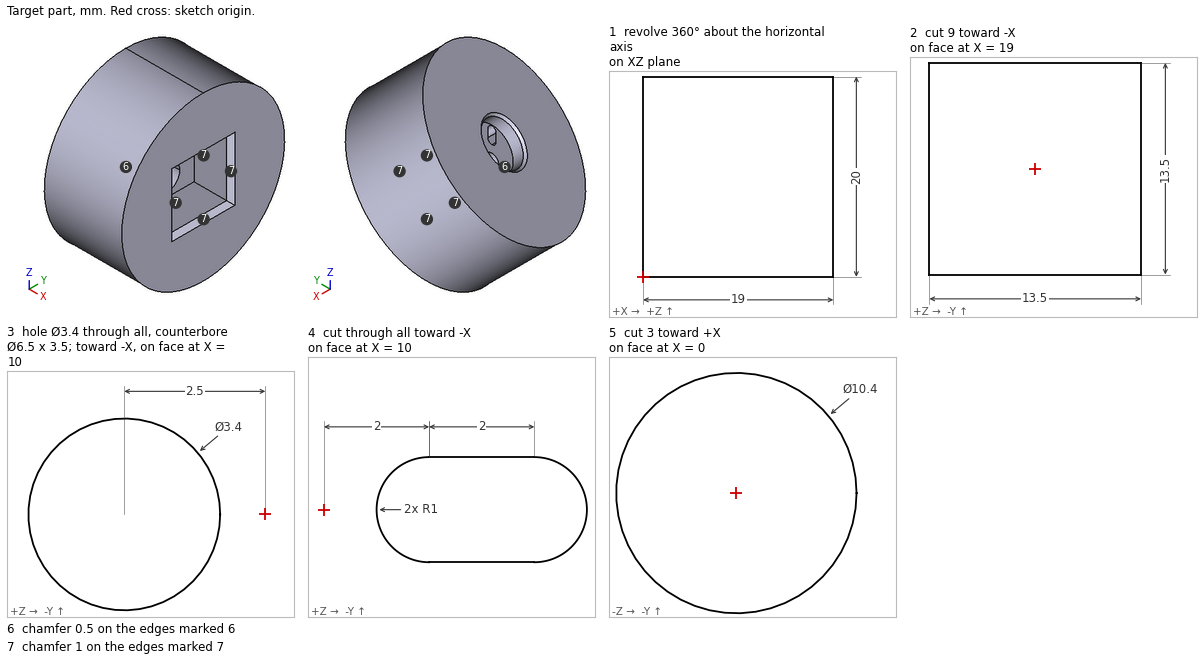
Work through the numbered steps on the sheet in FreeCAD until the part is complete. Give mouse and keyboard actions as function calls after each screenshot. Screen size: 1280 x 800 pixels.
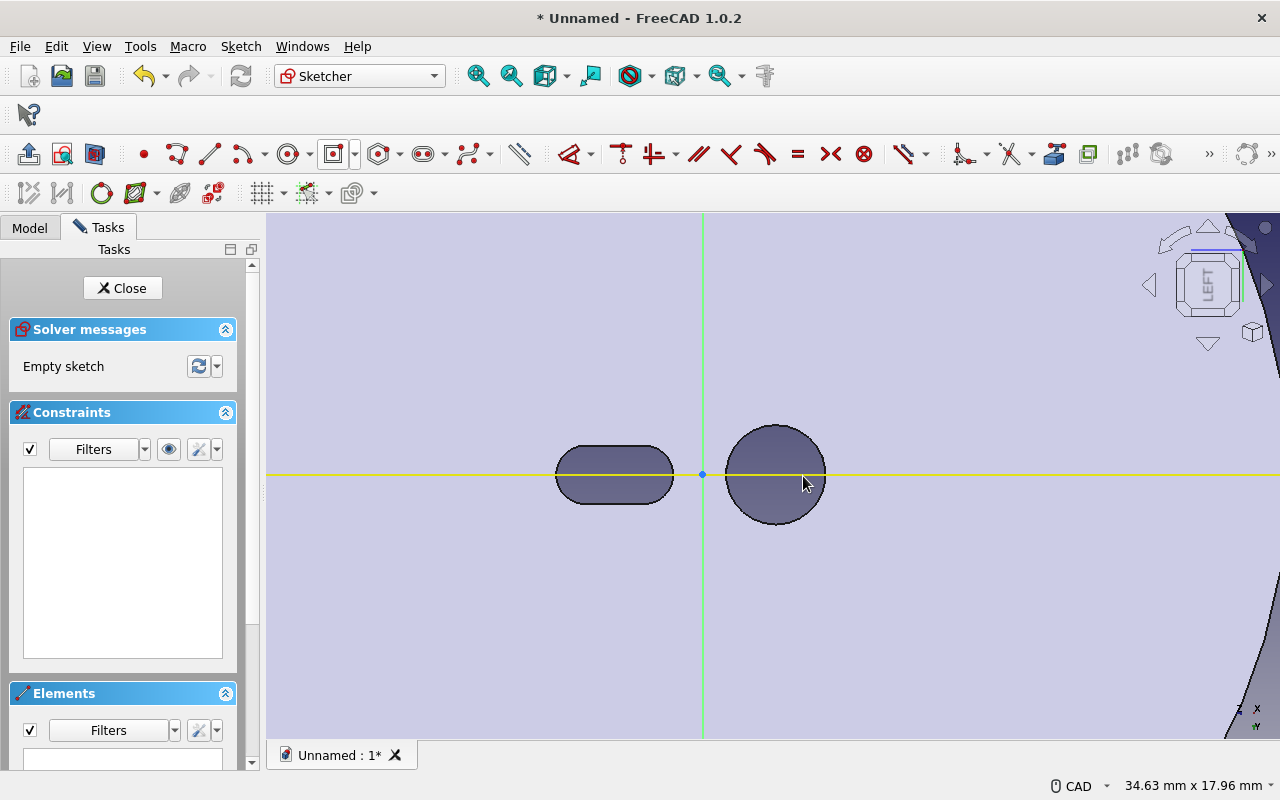
click(288, 154)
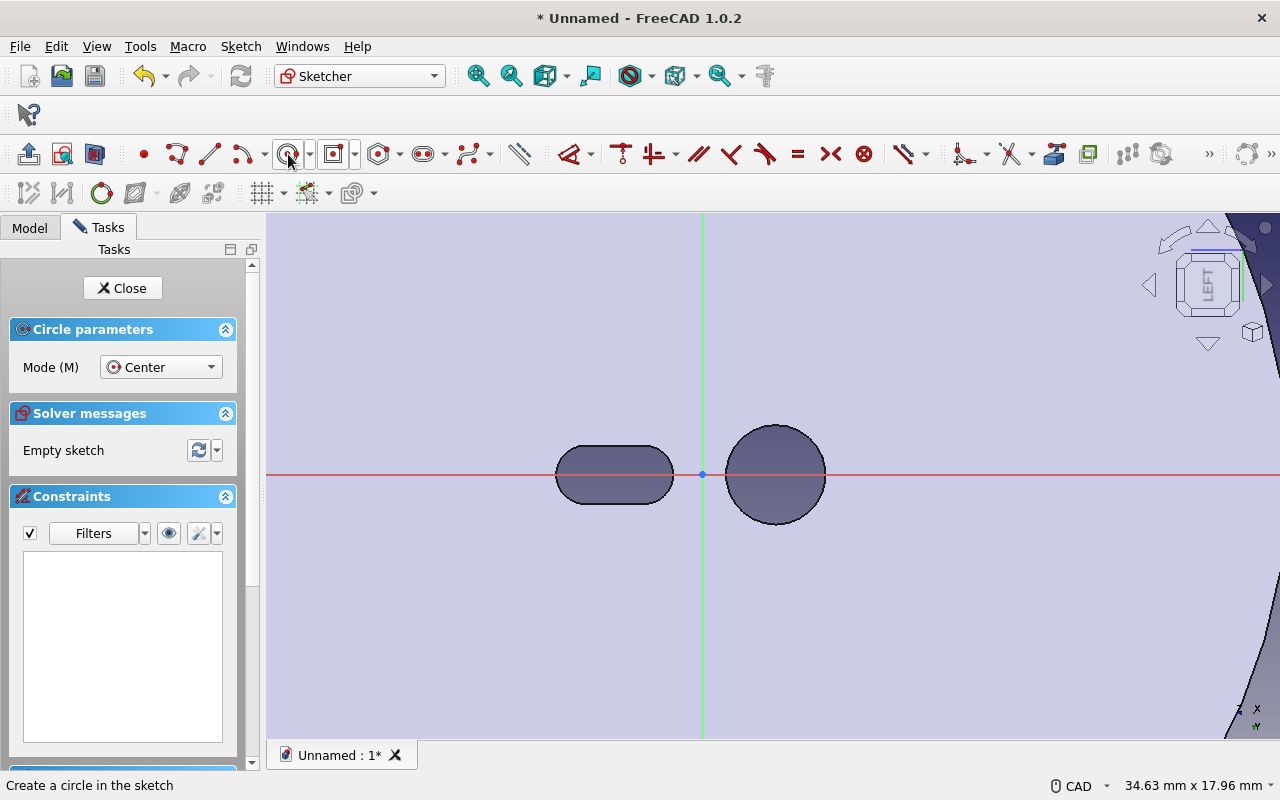
click(703, 475)
click(810, 367)
key(Escape)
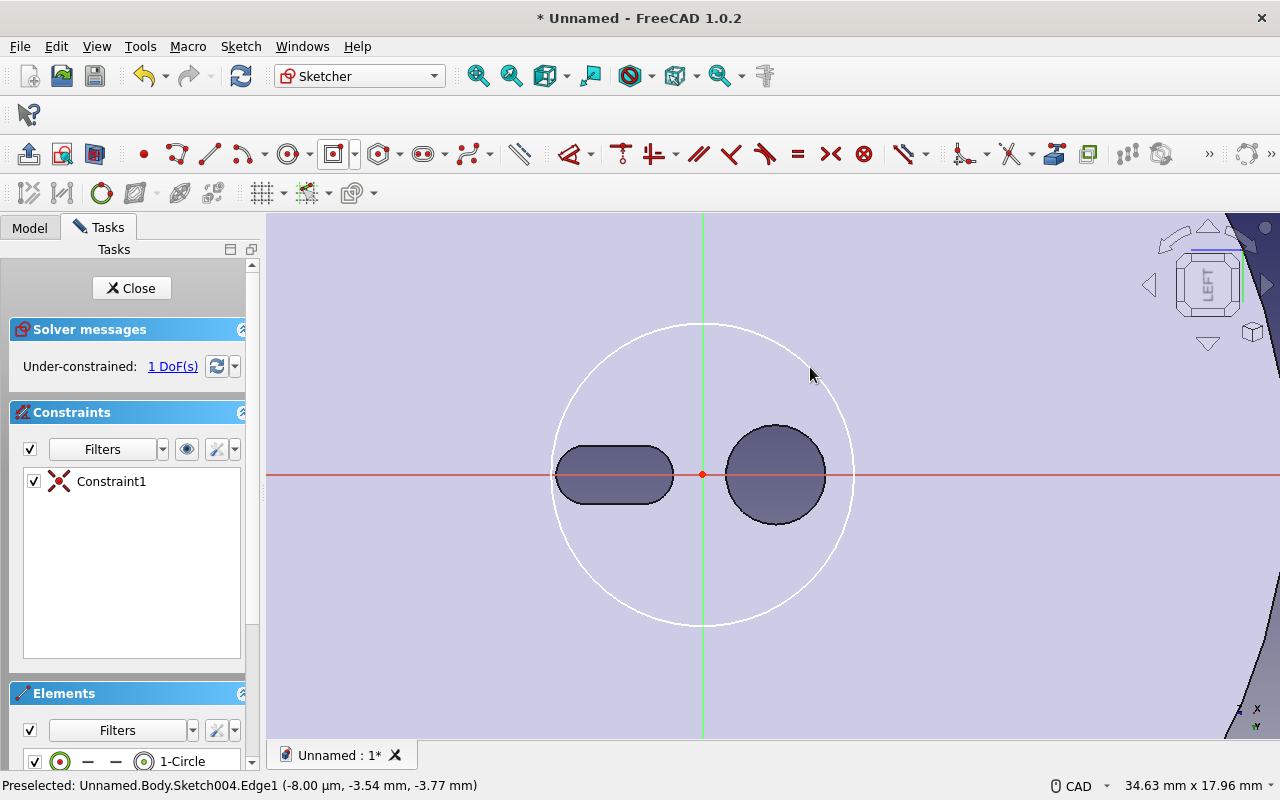
click(568, 154)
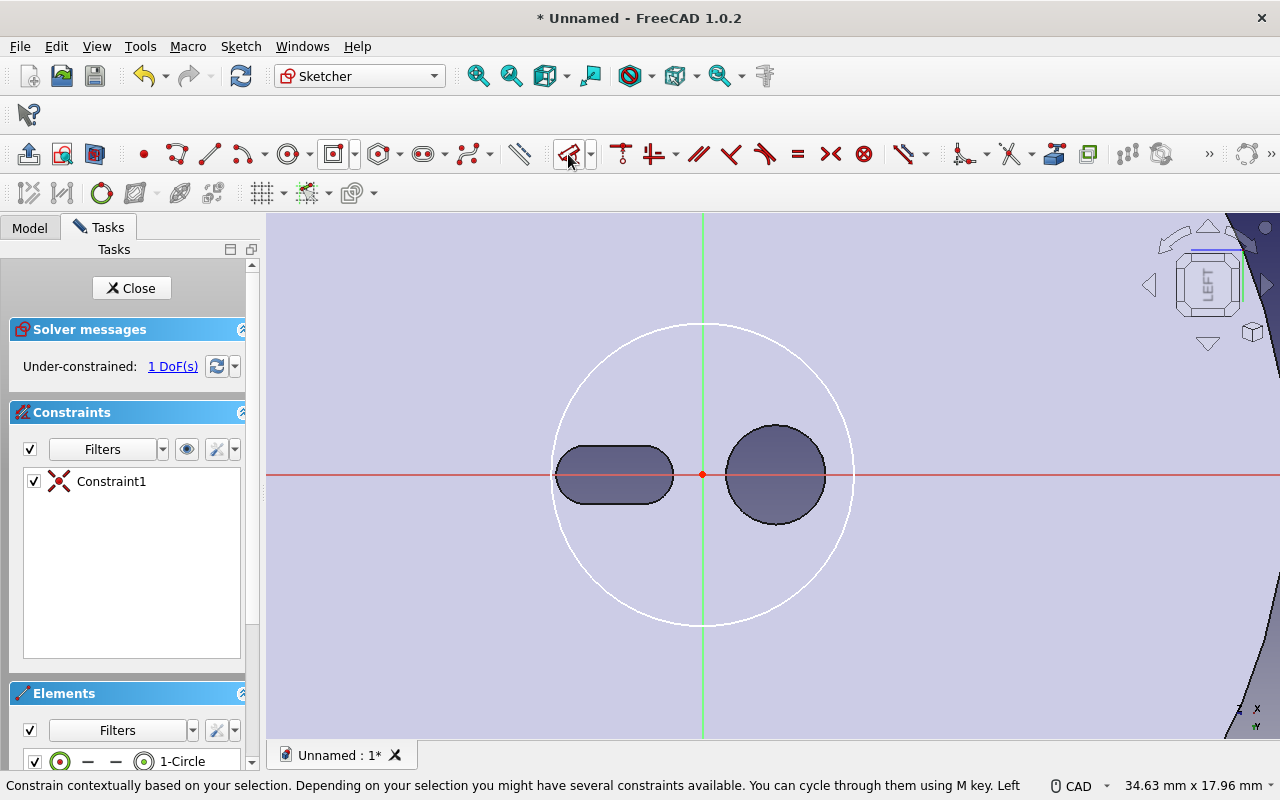
click(809, 367)
click(831, 344)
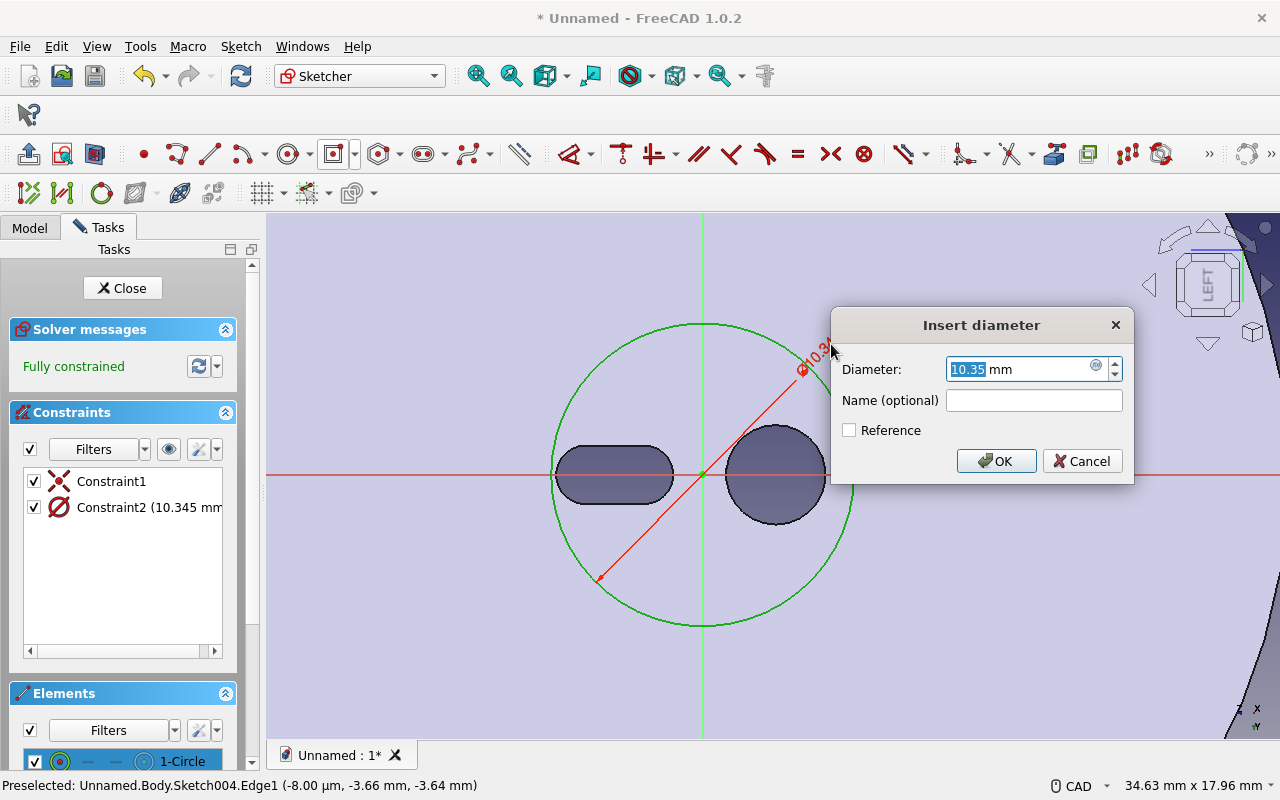
text(10.4)
key(Return)
key(Escape)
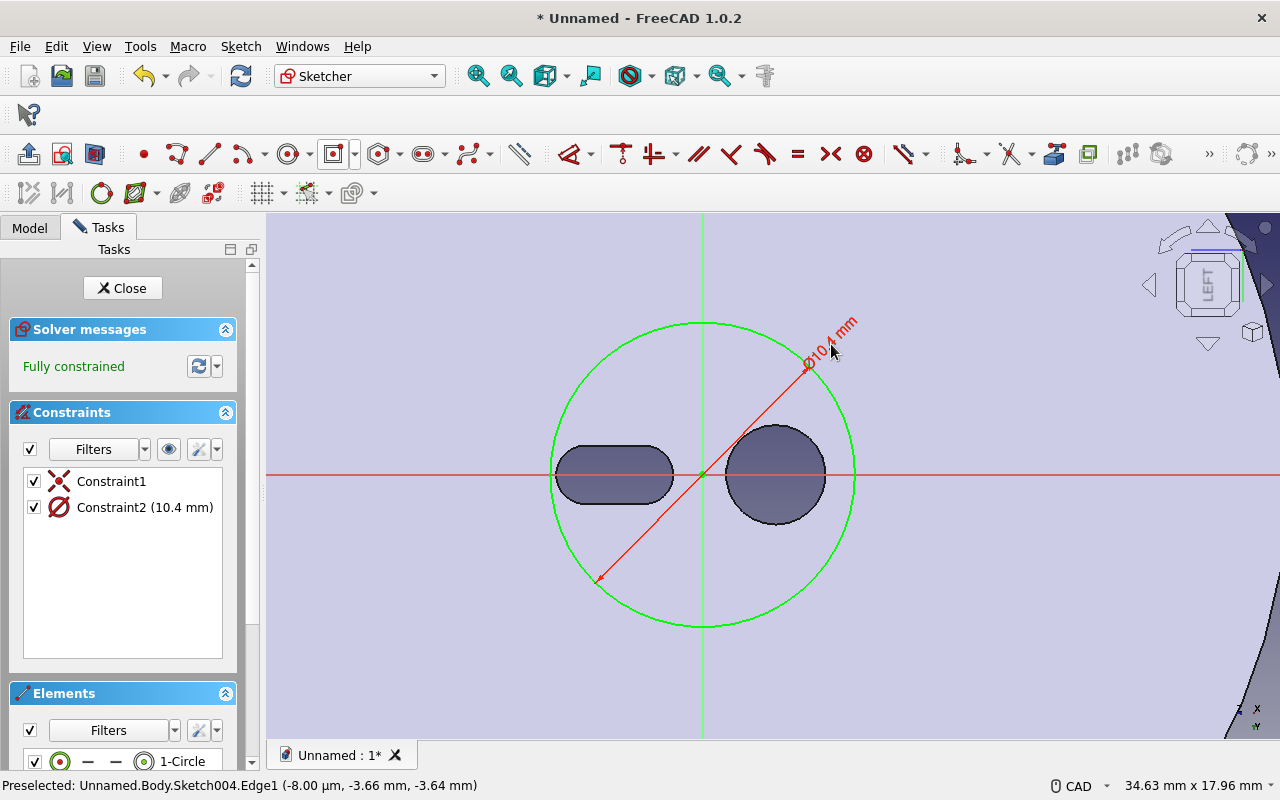
click(123, 288)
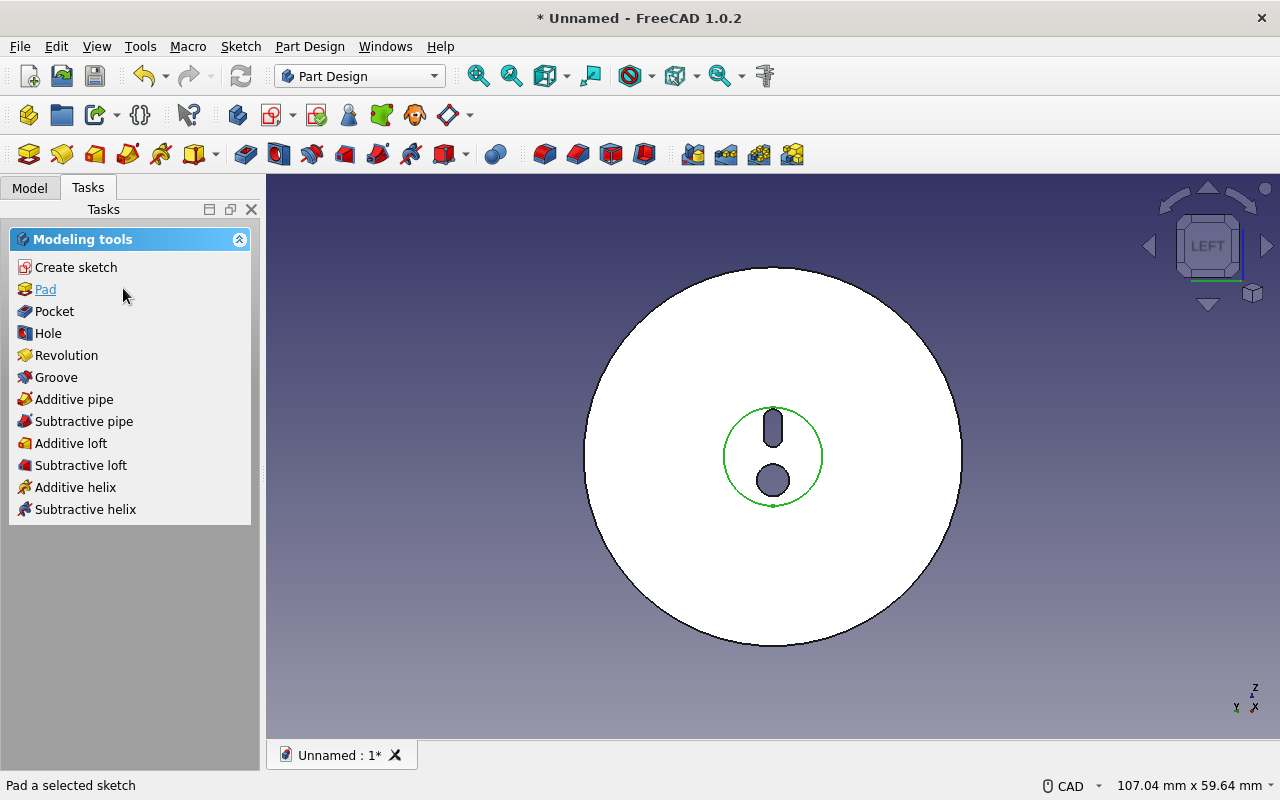
click(246, 154)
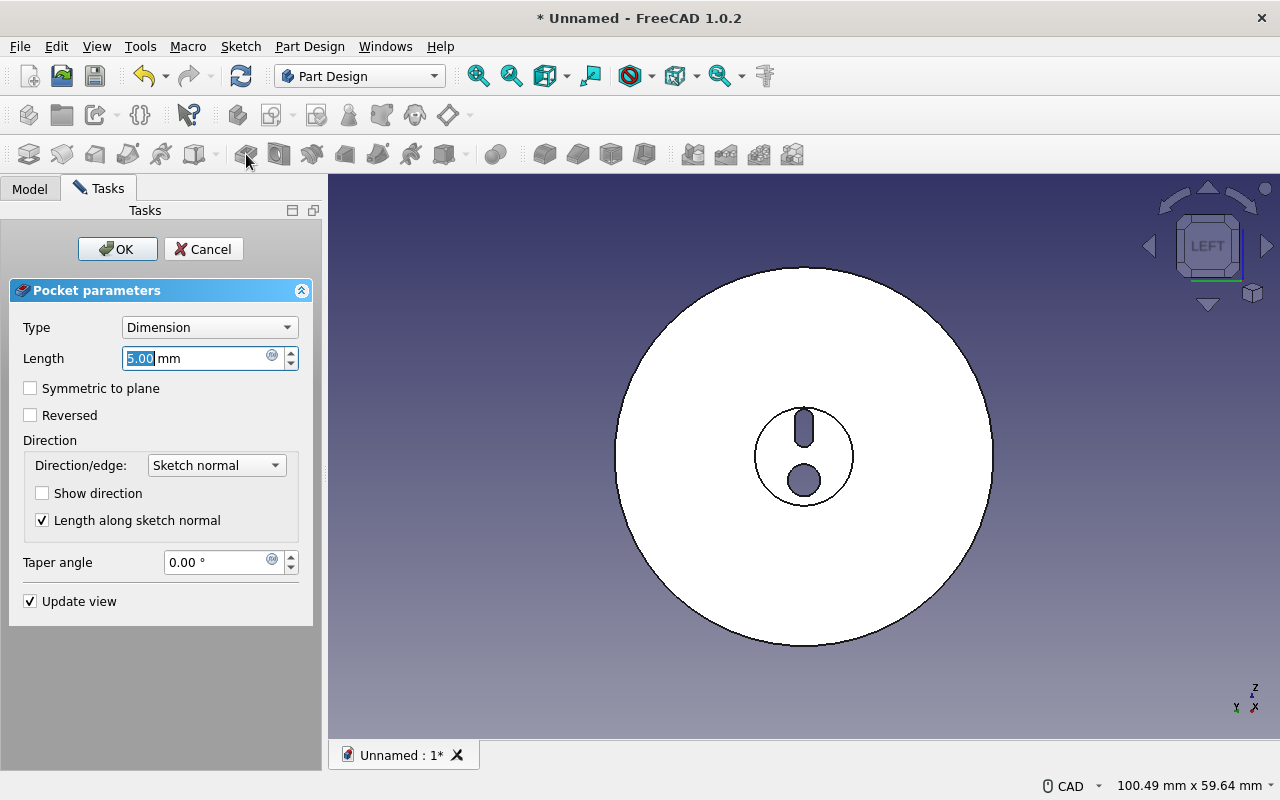
text(3)
key(Tab)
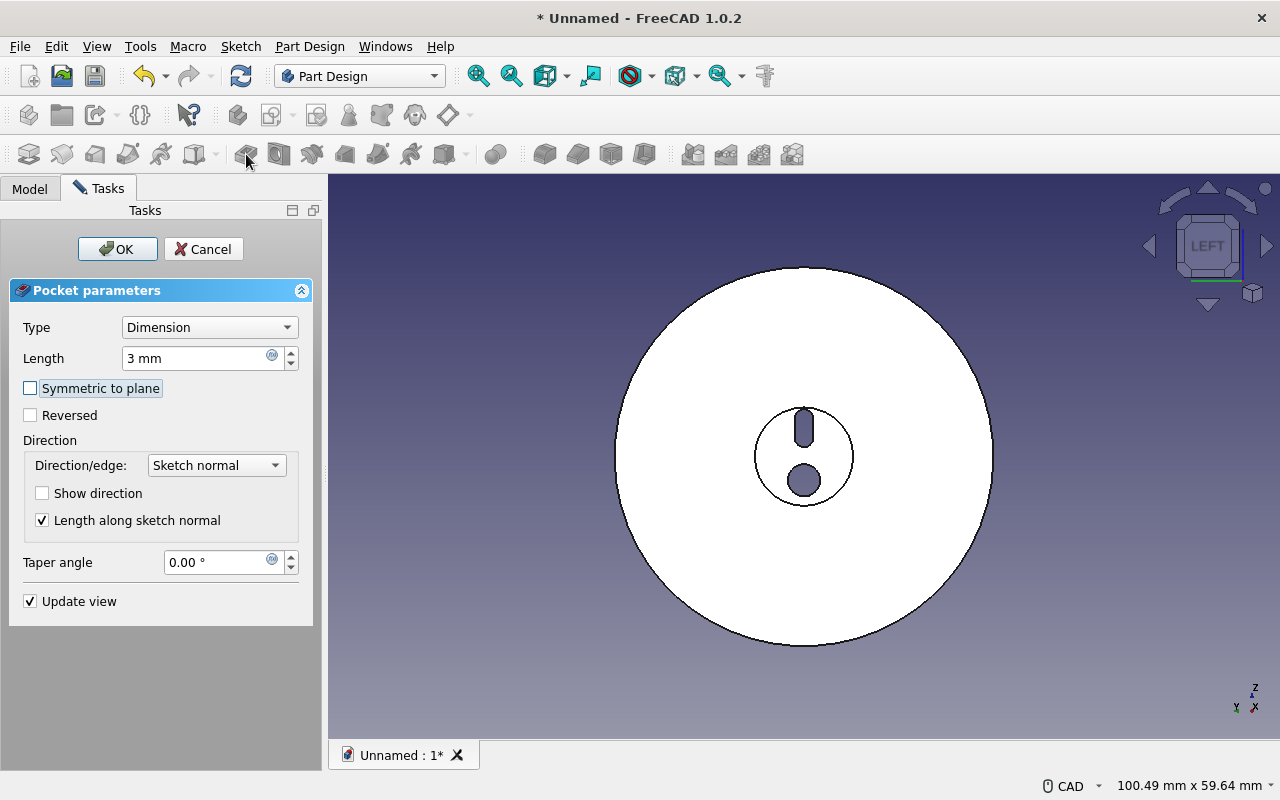
click(118, 249)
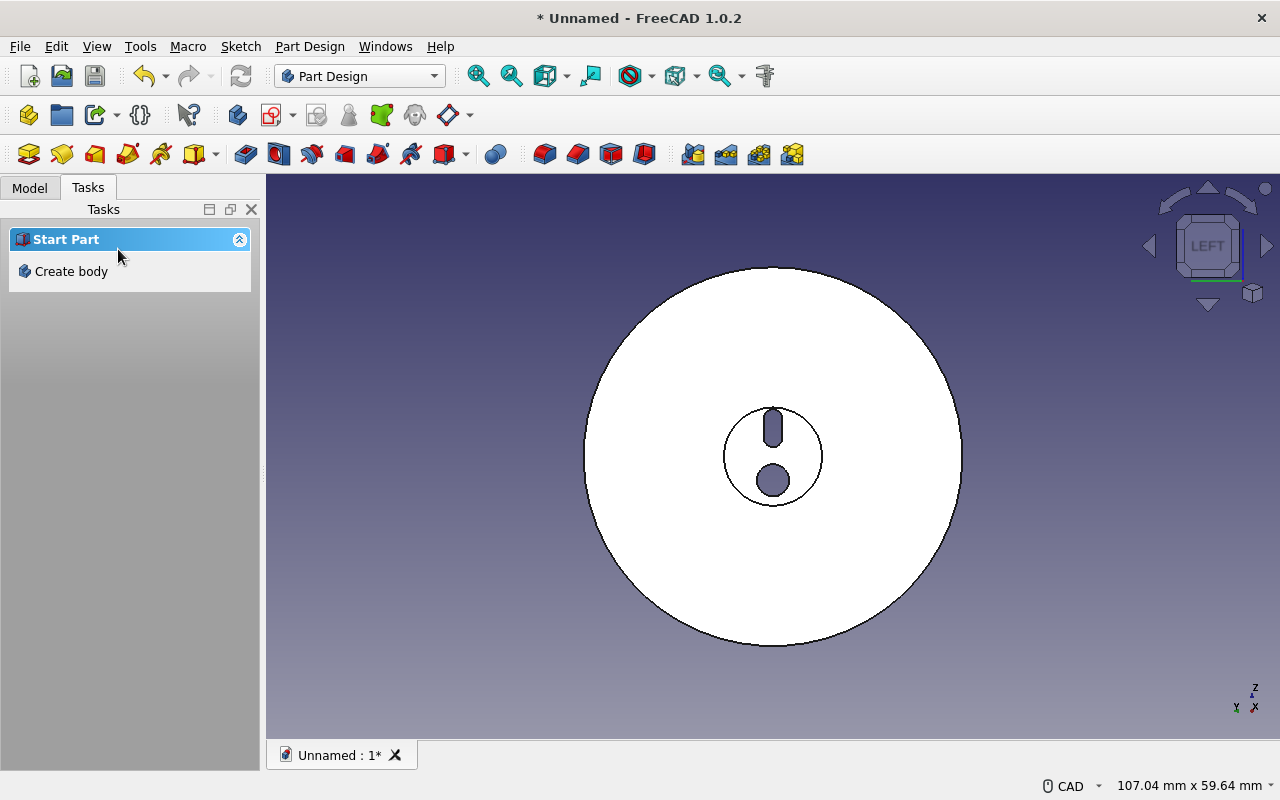
click(773, 406)